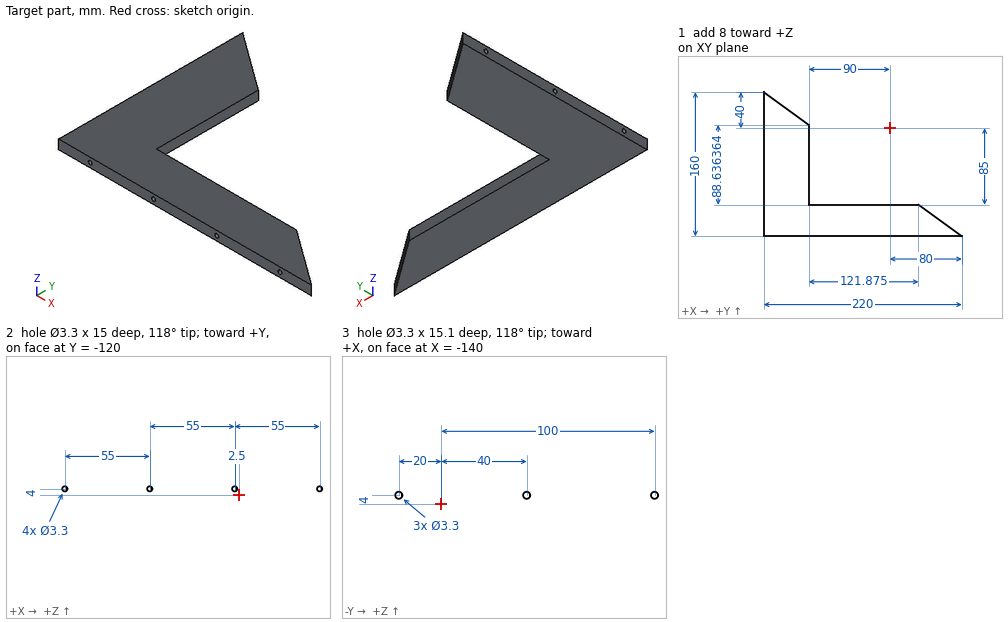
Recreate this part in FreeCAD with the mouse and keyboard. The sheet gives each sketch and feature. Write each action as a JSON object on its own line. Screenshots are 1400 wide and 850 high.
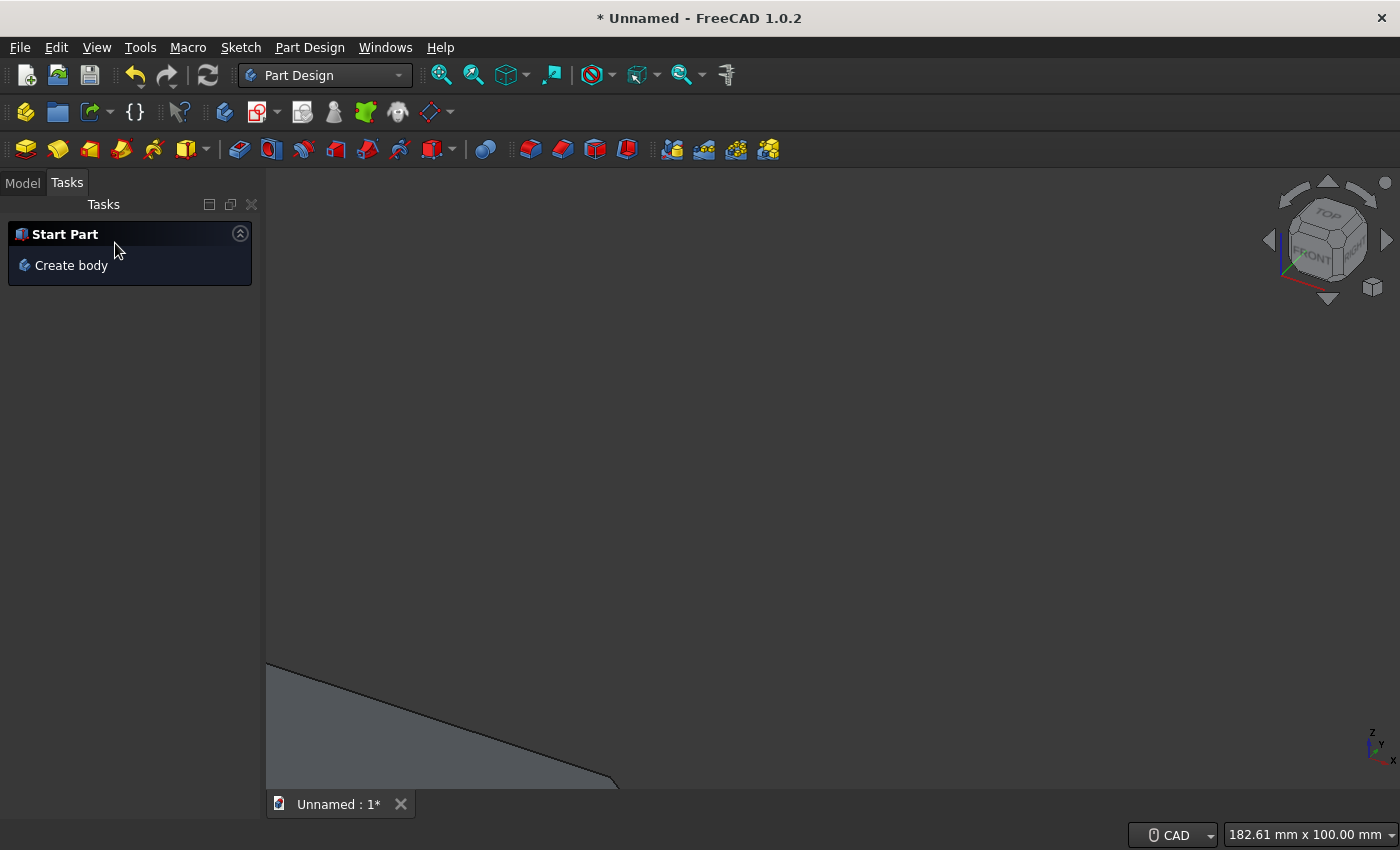
{"action": "key", "text": "v f"}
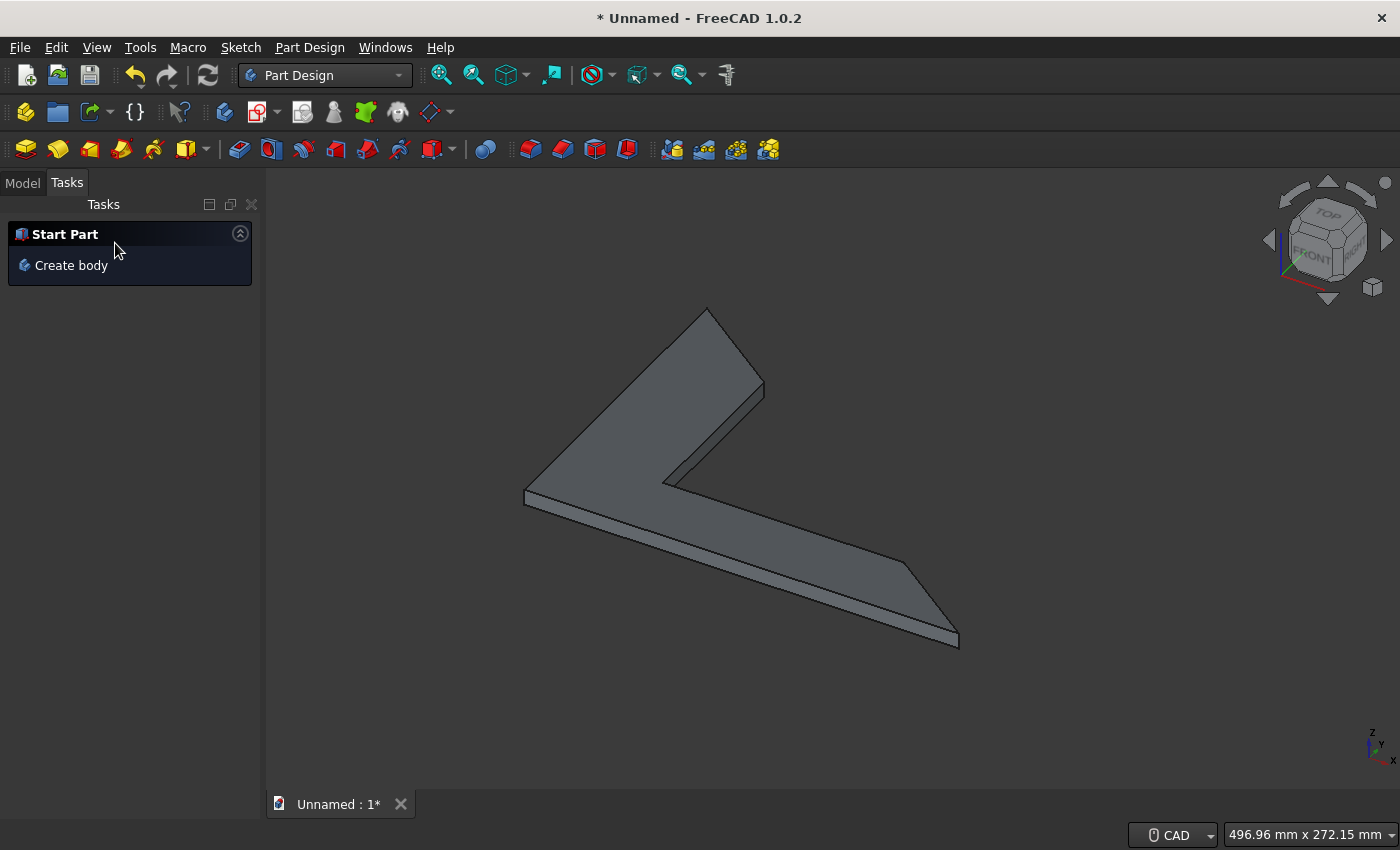
{"action": "key", "text": "0"}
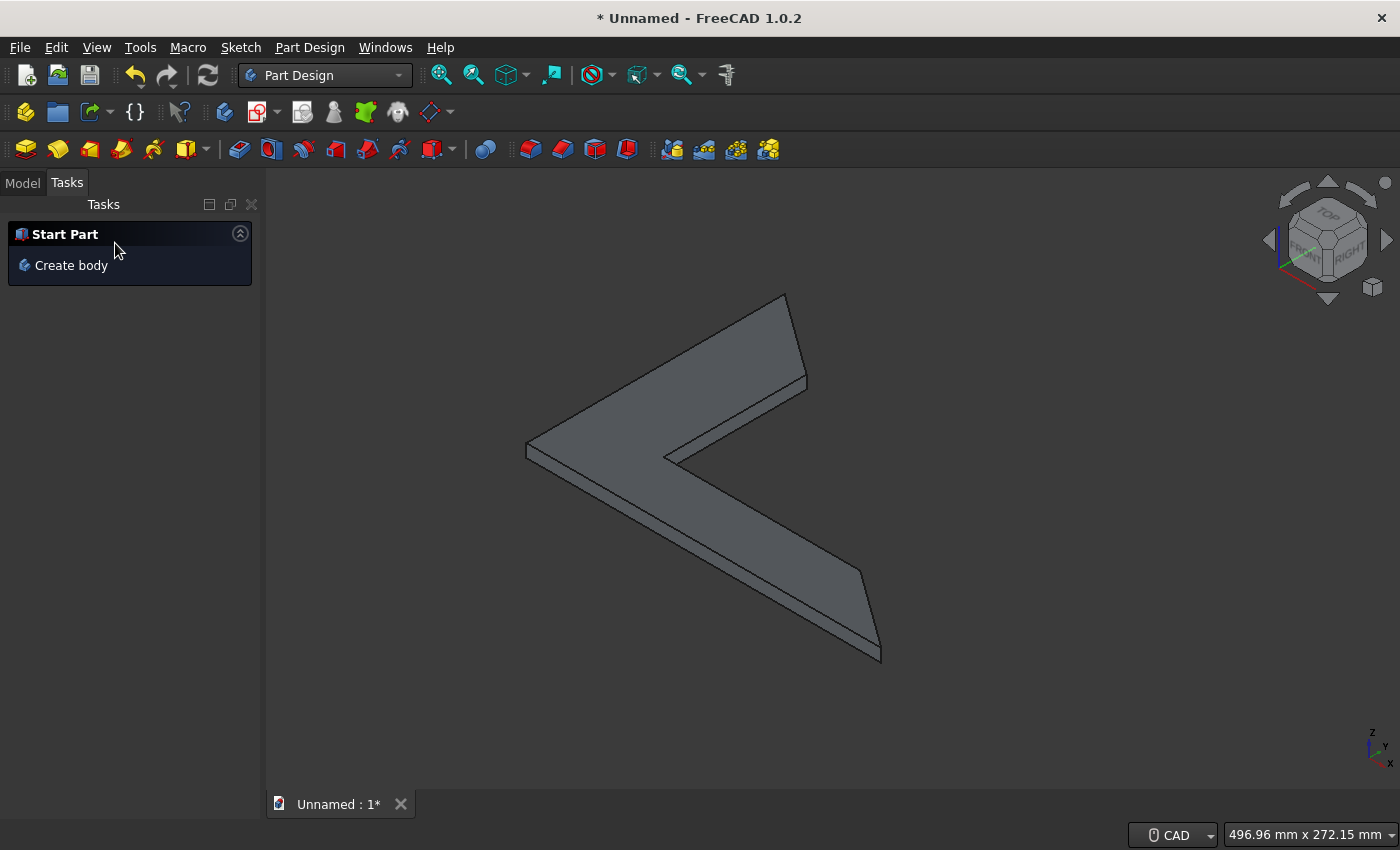
{"action": "key", "text": "1"}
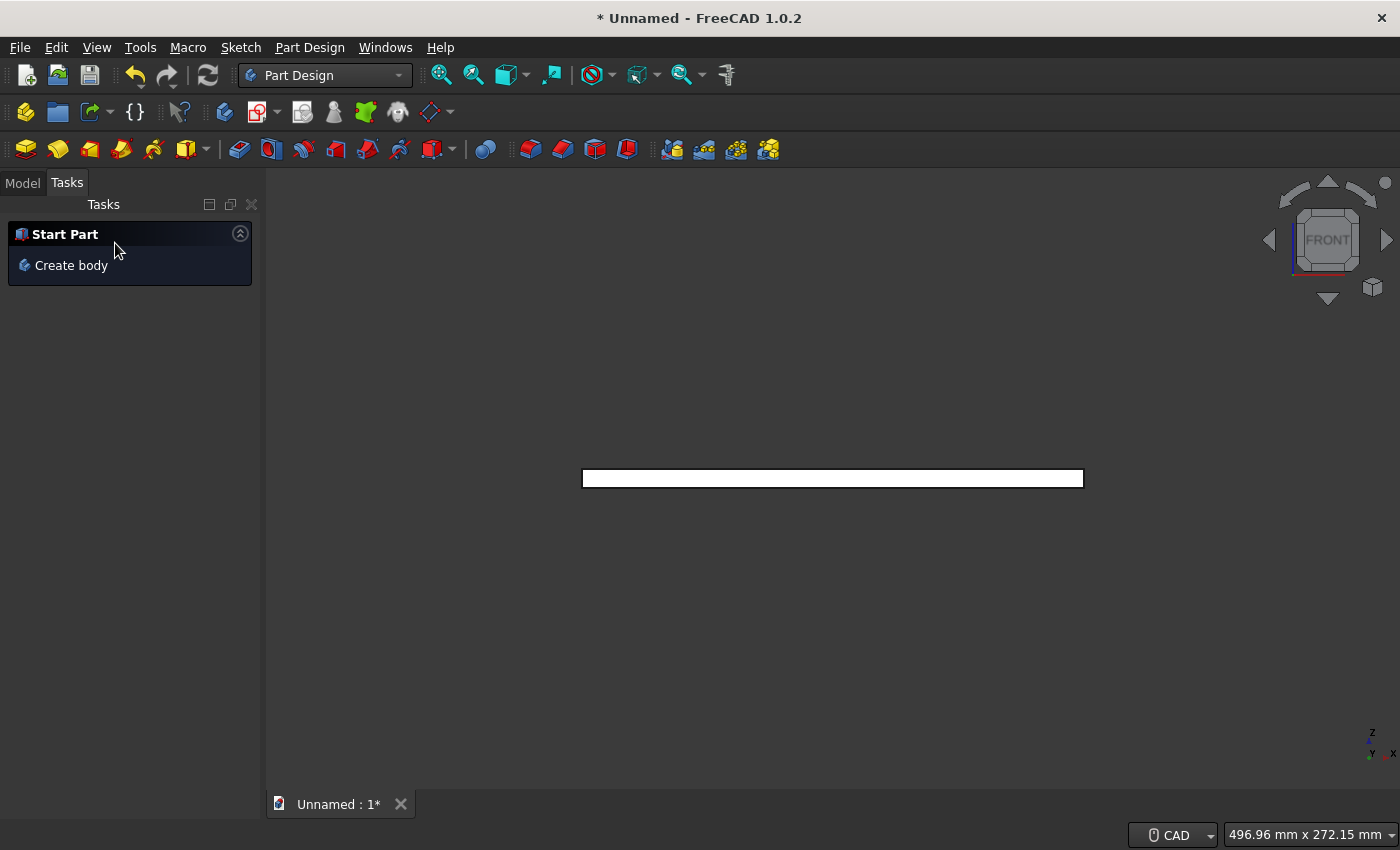
{"action": "left_click", "coordinate": [442, 76]}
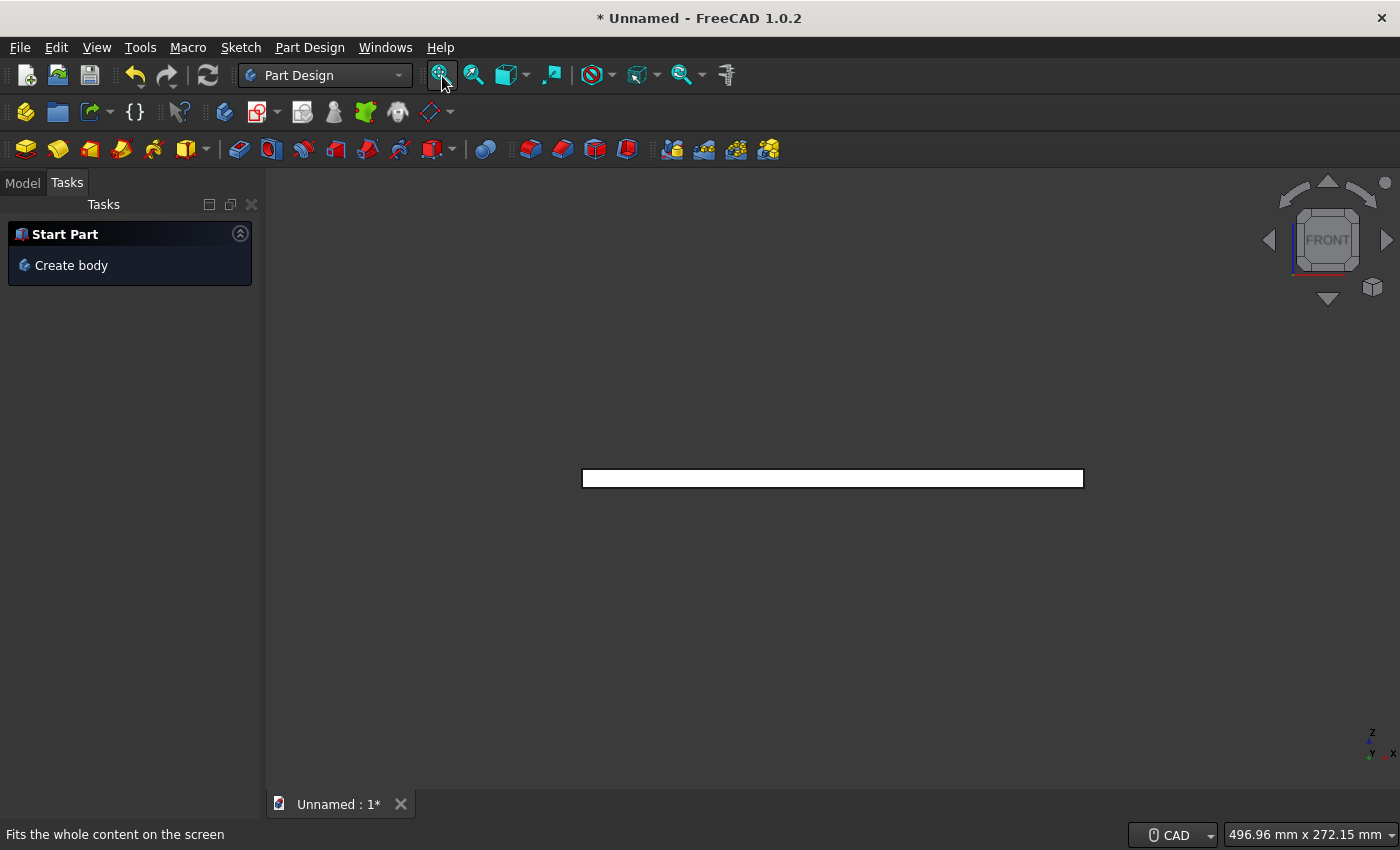
{"action": "left_click", "coordinate": [1048, 478]}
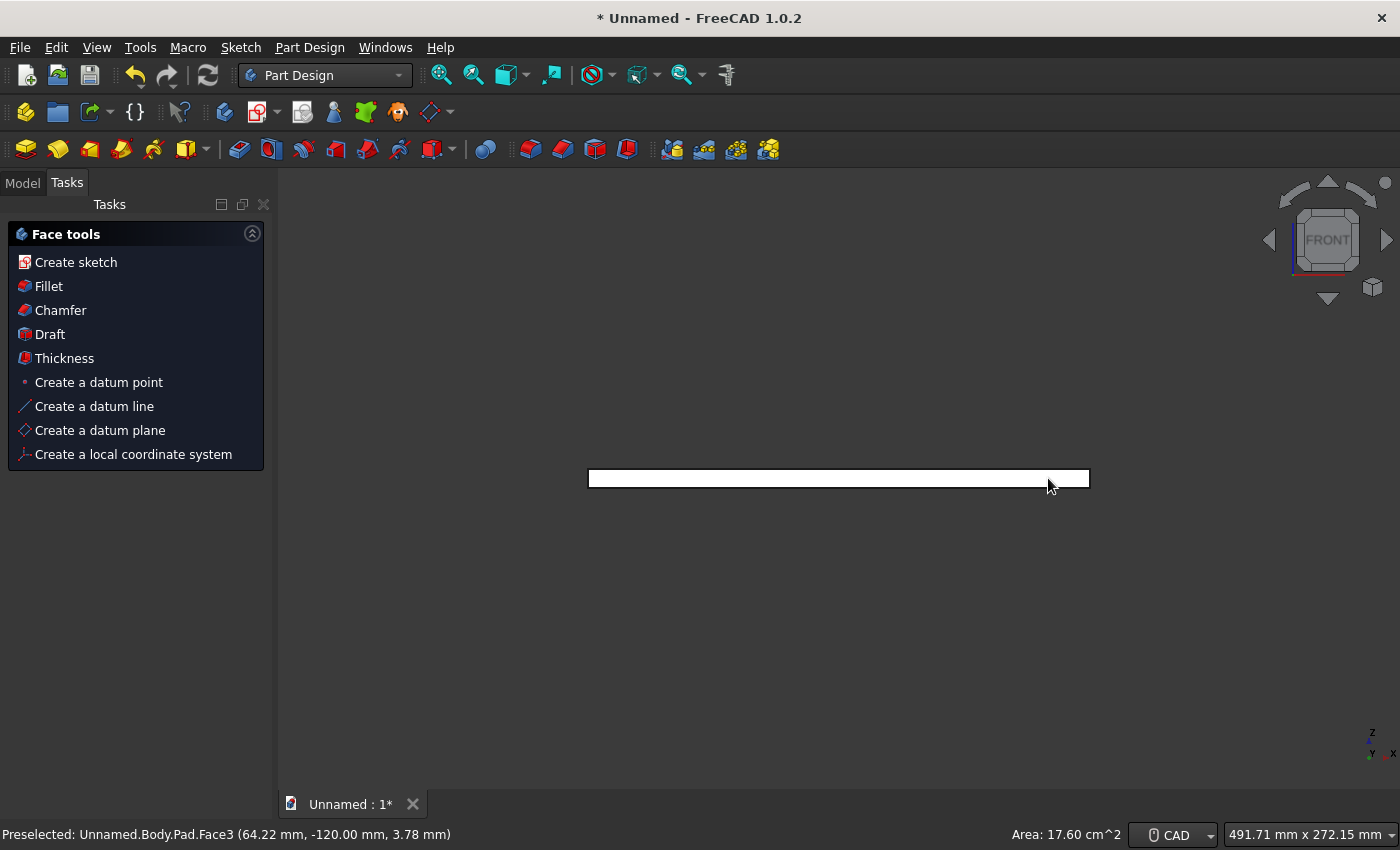
{"action": "left_click", "coordinate": [258, 112]}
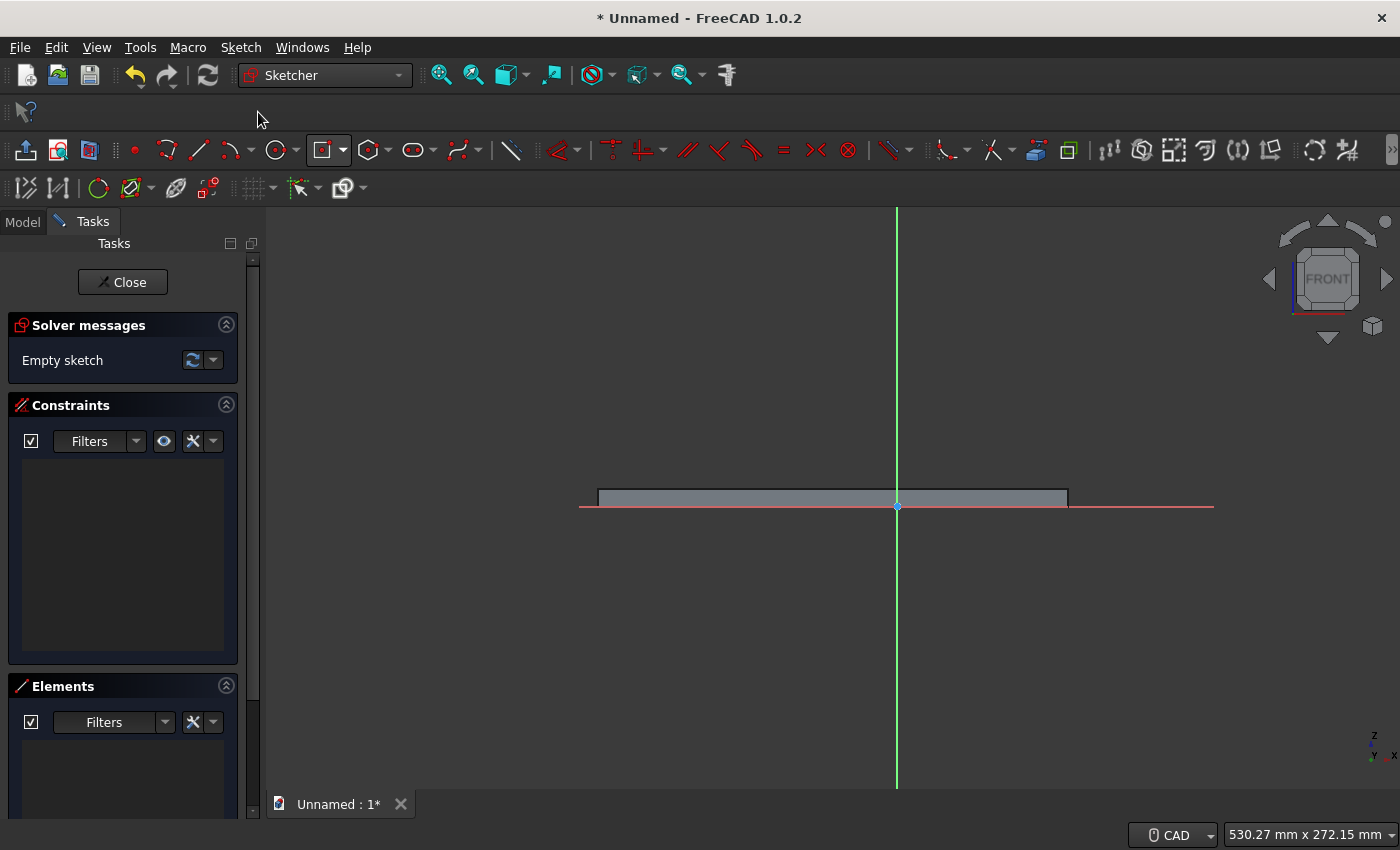
{"action": "scroll", "coordinate": [916, 504], "scroll_direction": "up", "scroll_amount": 3}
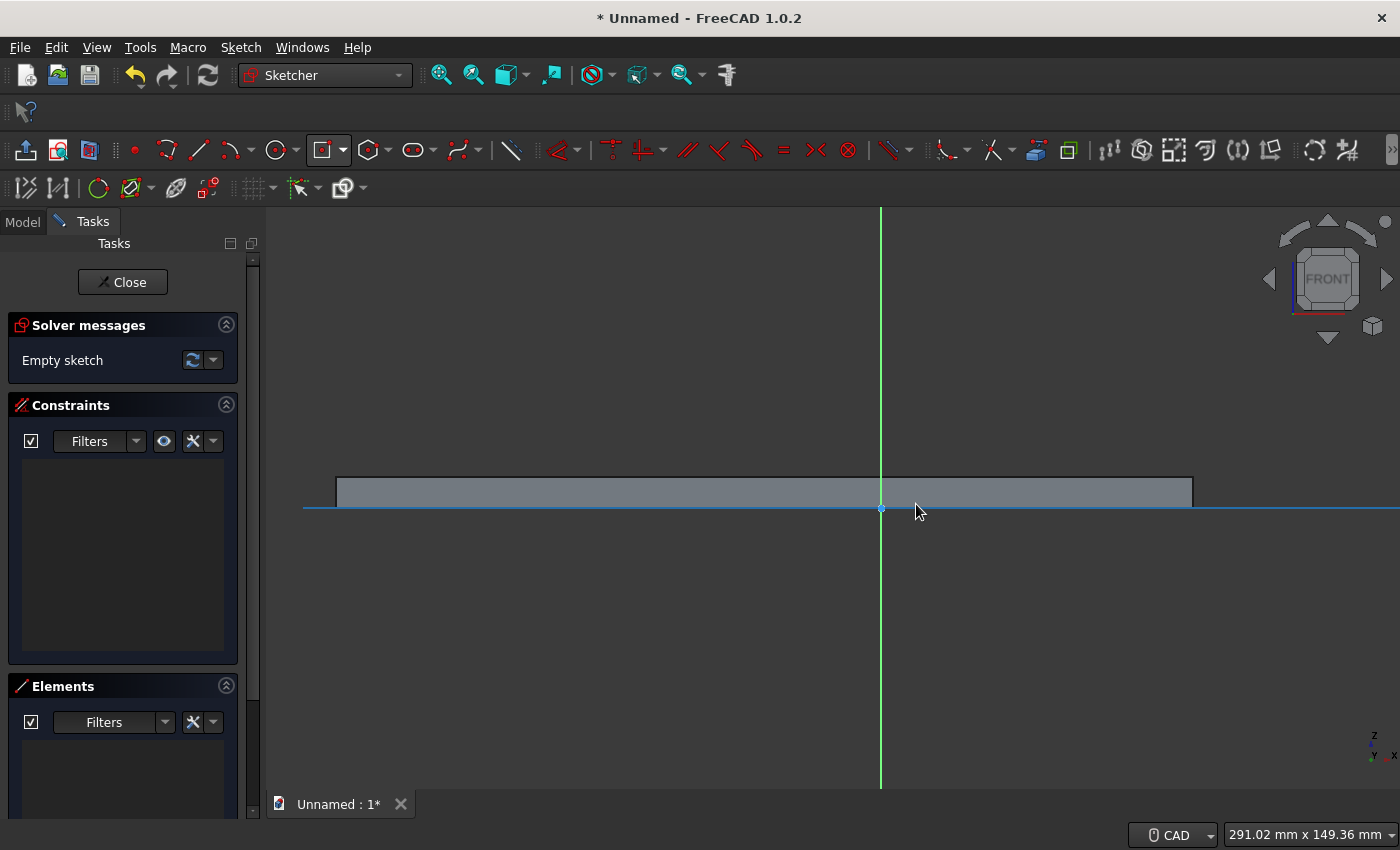
{"action": "key", "text": "g c"}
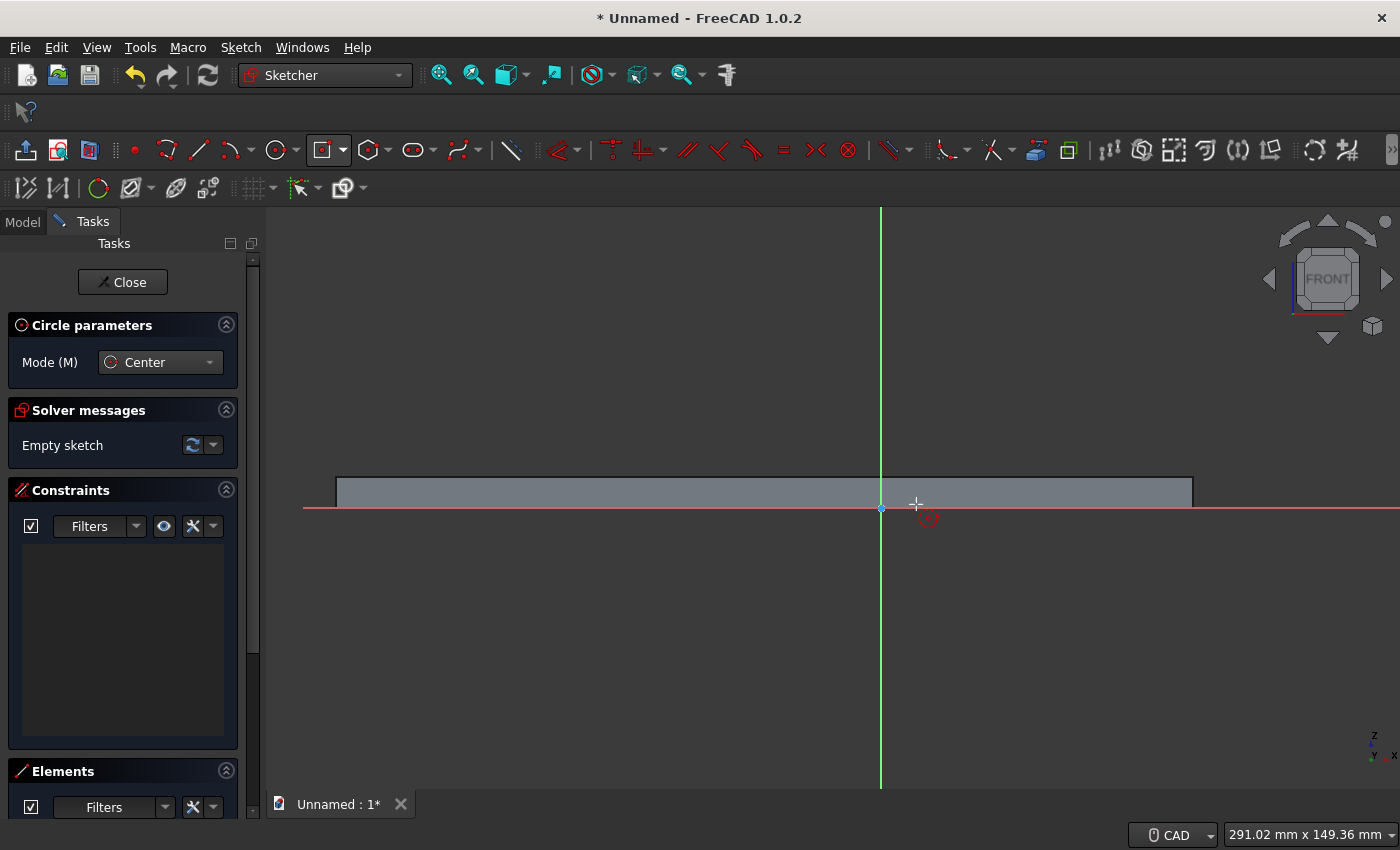
{"action": "scroll", "coordinate": [443, 493], "scroll_direction": "up", "scroll_amount": 7}